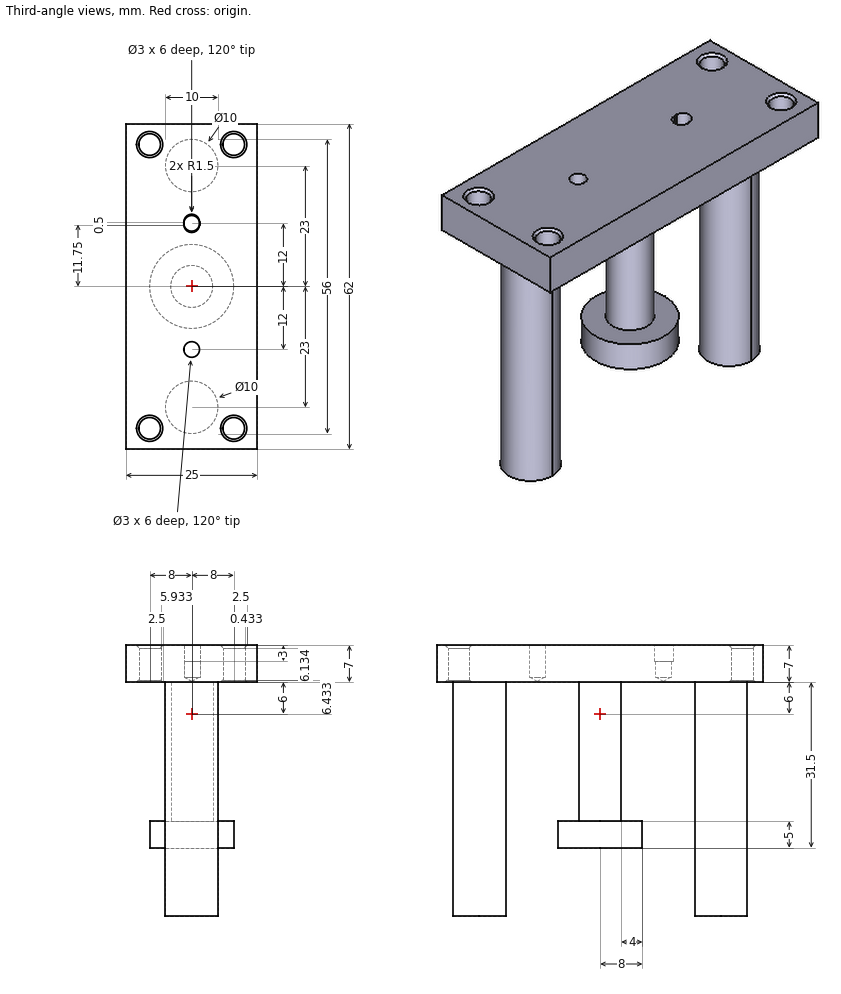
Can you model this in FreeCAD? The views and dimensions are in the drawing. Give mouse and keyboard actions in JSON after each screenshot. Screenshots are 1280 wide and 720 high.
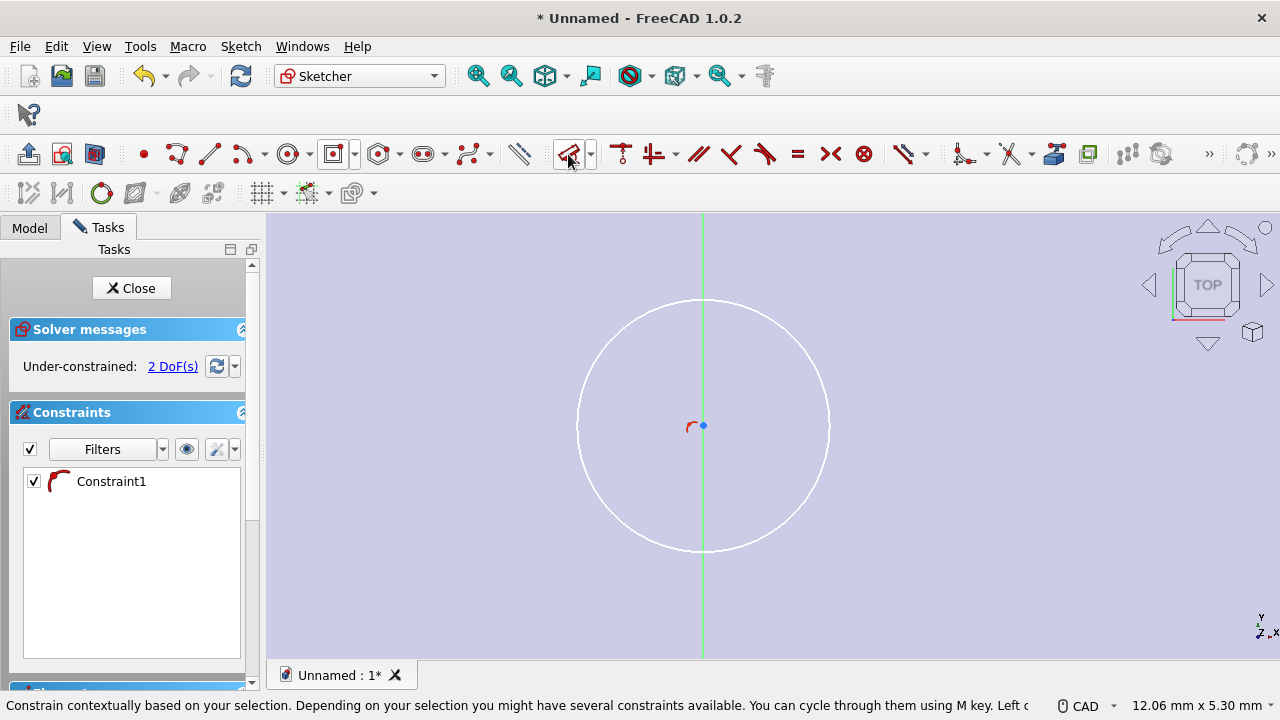
{"action": "left_click", "coordinate": [792, 336]}
{"action": "left_click", "coordinate": [814, 313]}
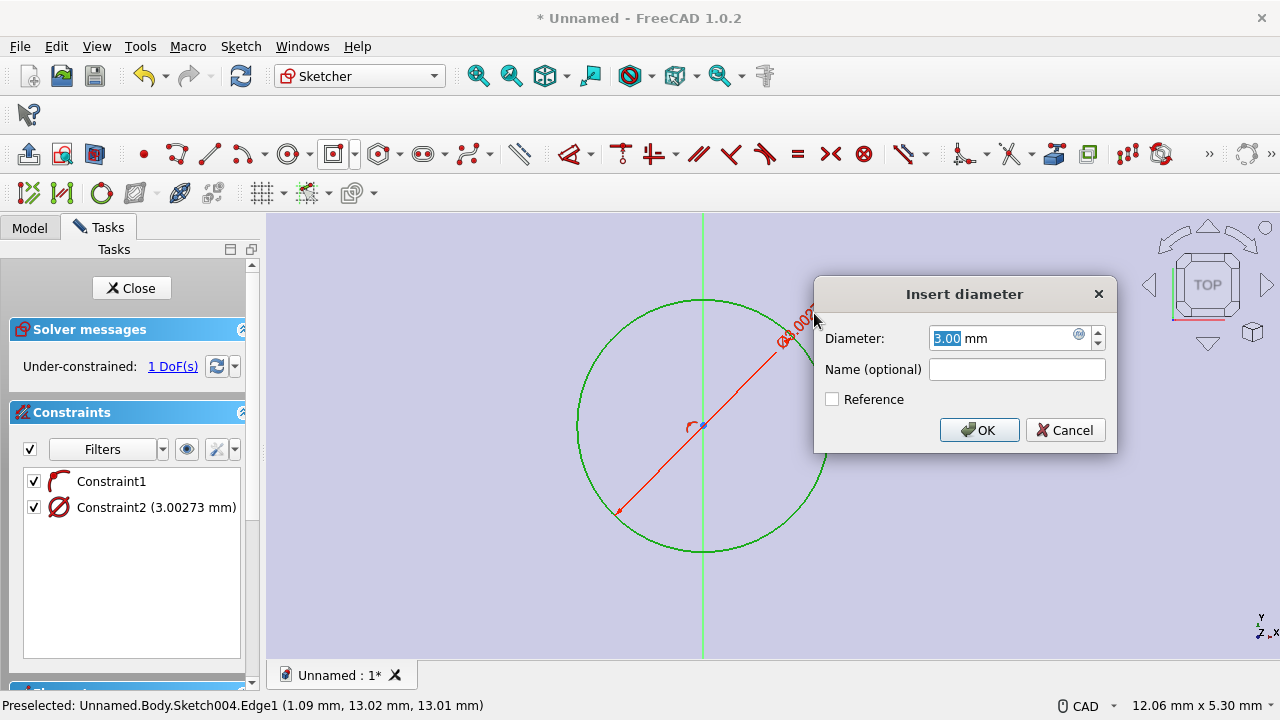
{"action": "type", "text": "3"}
{"action": "key", "text": "Return"}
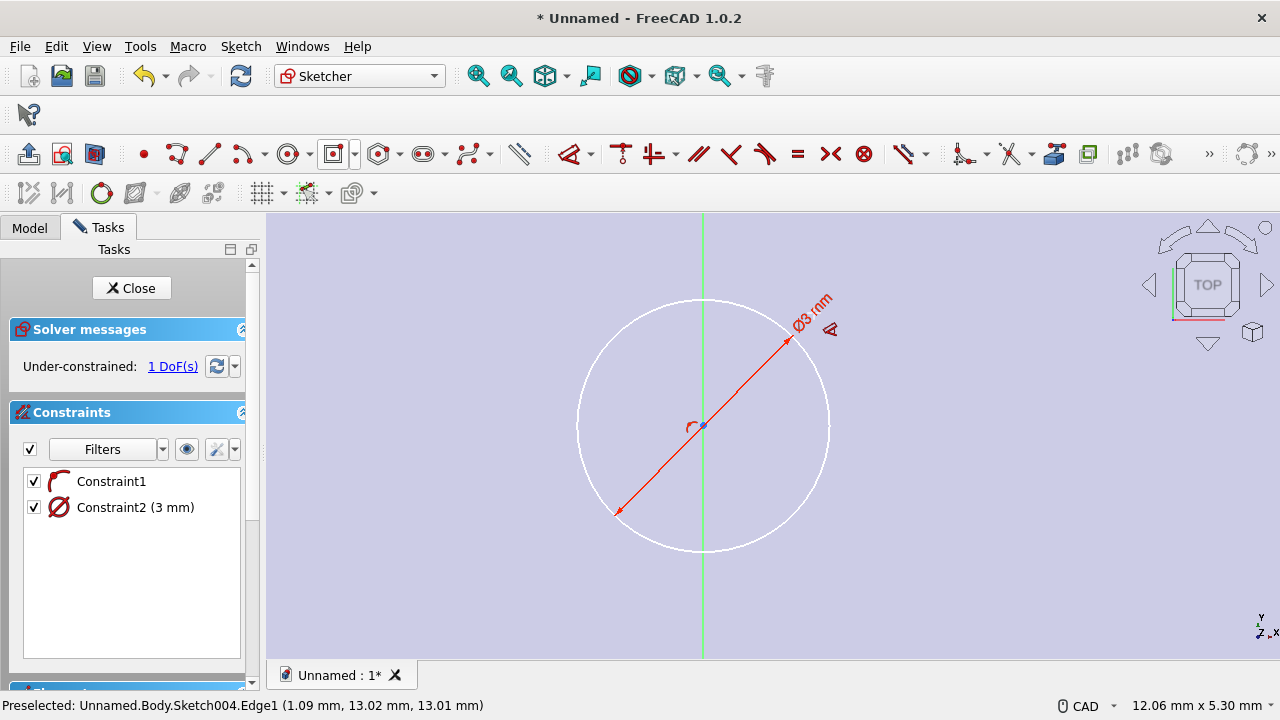
{"action": "left_click", "coordinate": [703, 426]}
{"action": "left_click", "coordinate": [737, 529]}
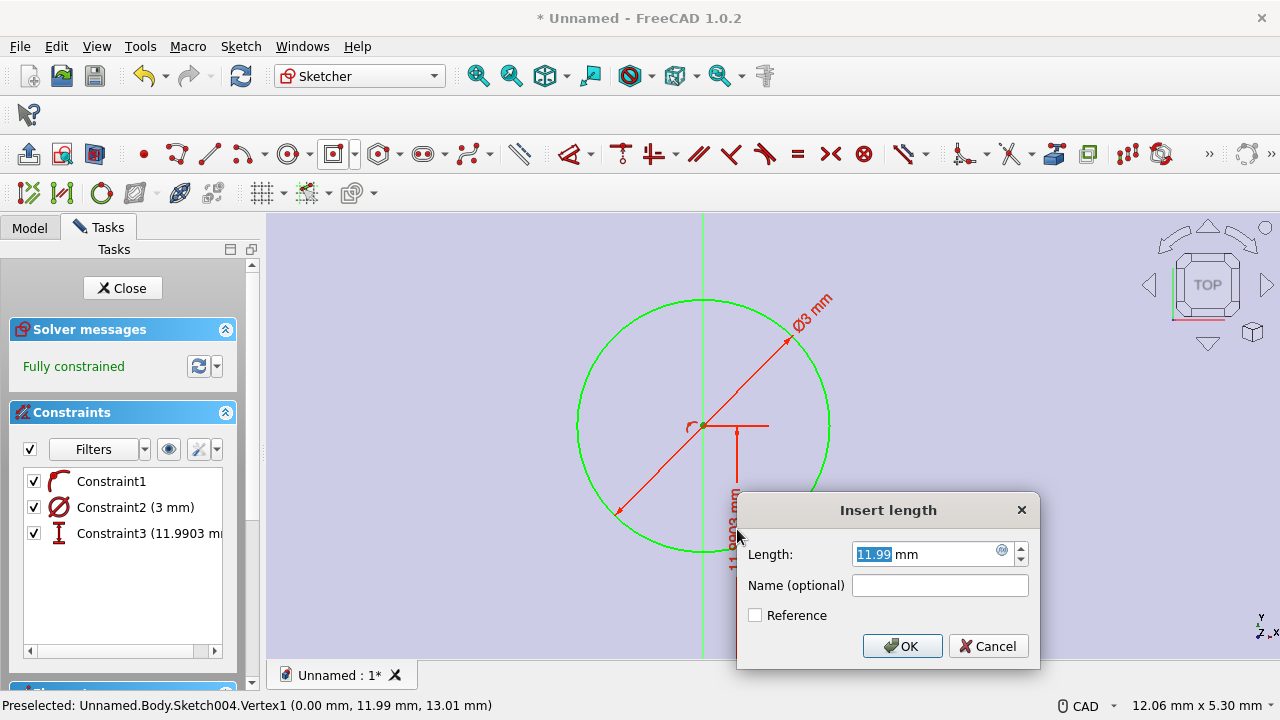
{"action": "type", "text": "12"}
{"action": "key", "text": "Return"}
{"action": "key", "text": "Escape"}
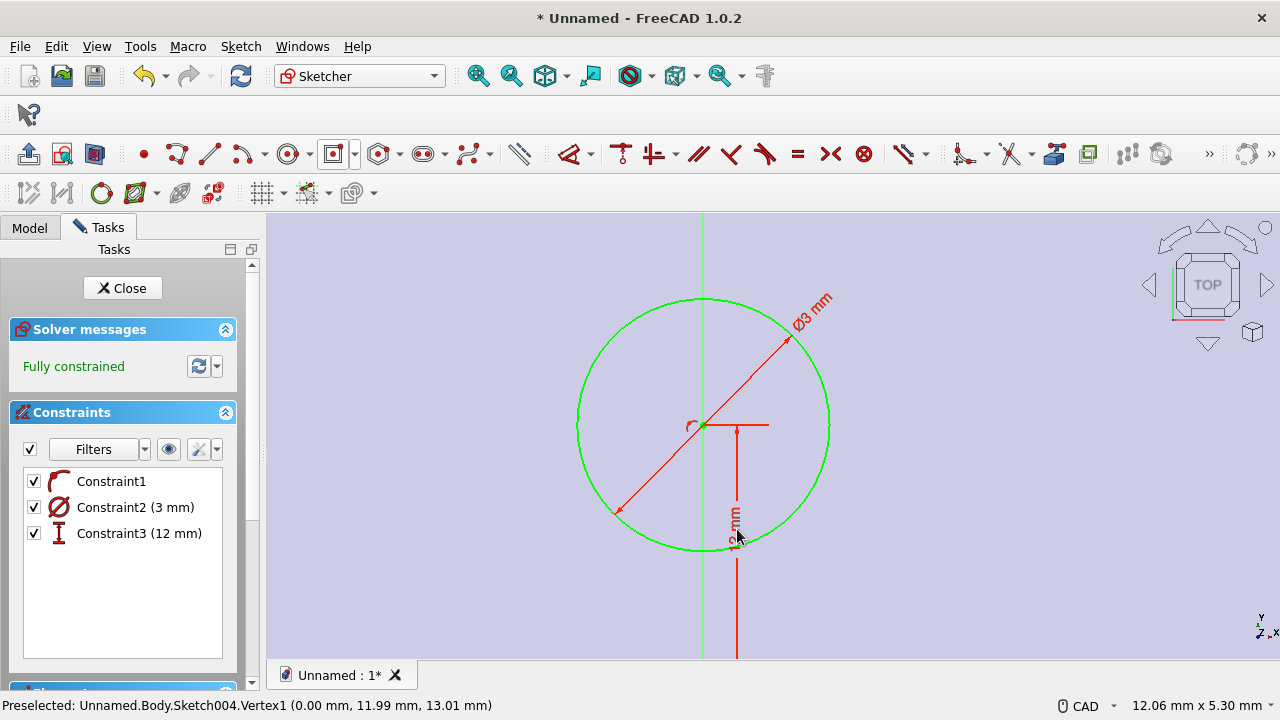
{"action": "left_click", "coordinate": [123, 288]}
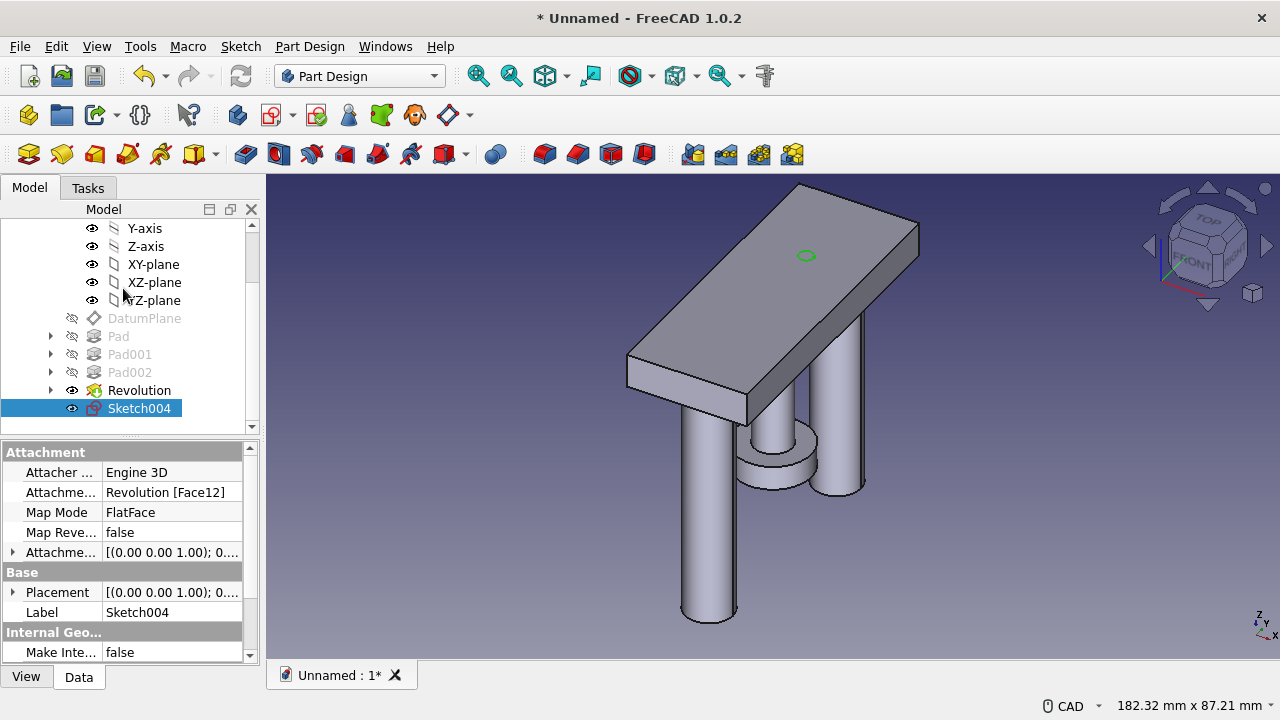
{"action": "left_click", "coordinate": [279, 154]}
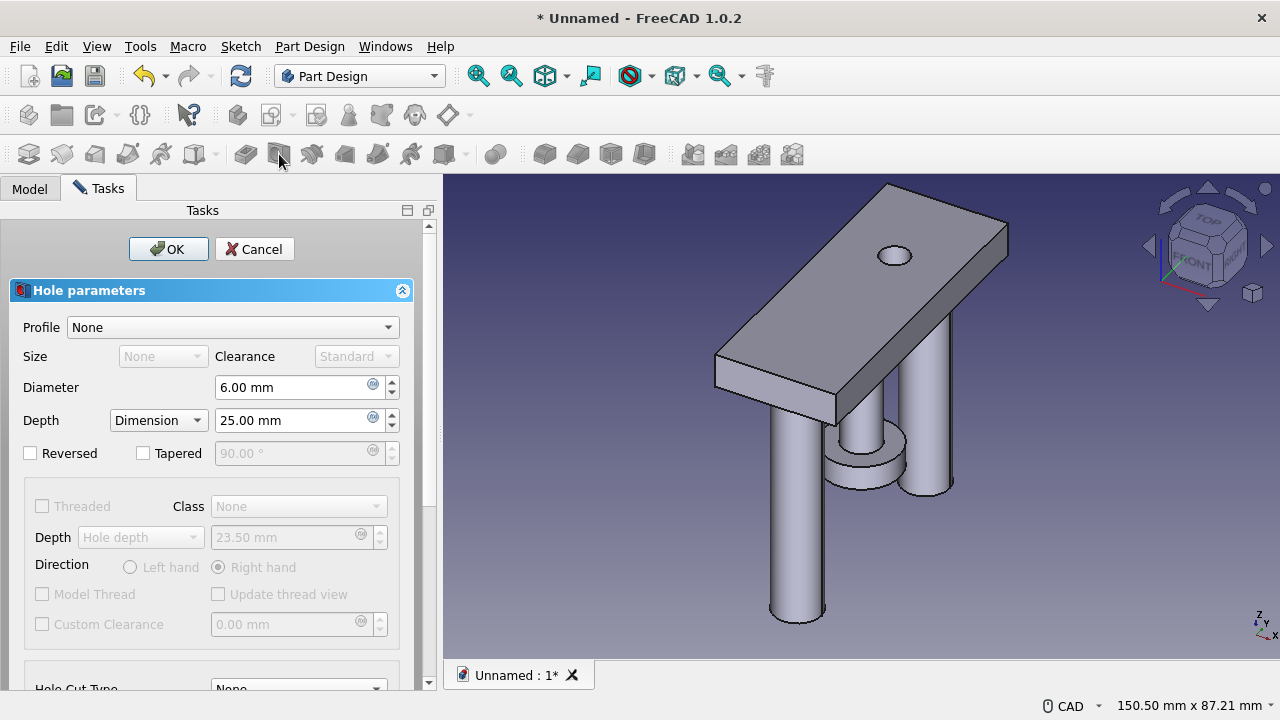
{"action": "triple_click", "coordinate": [300, 388]}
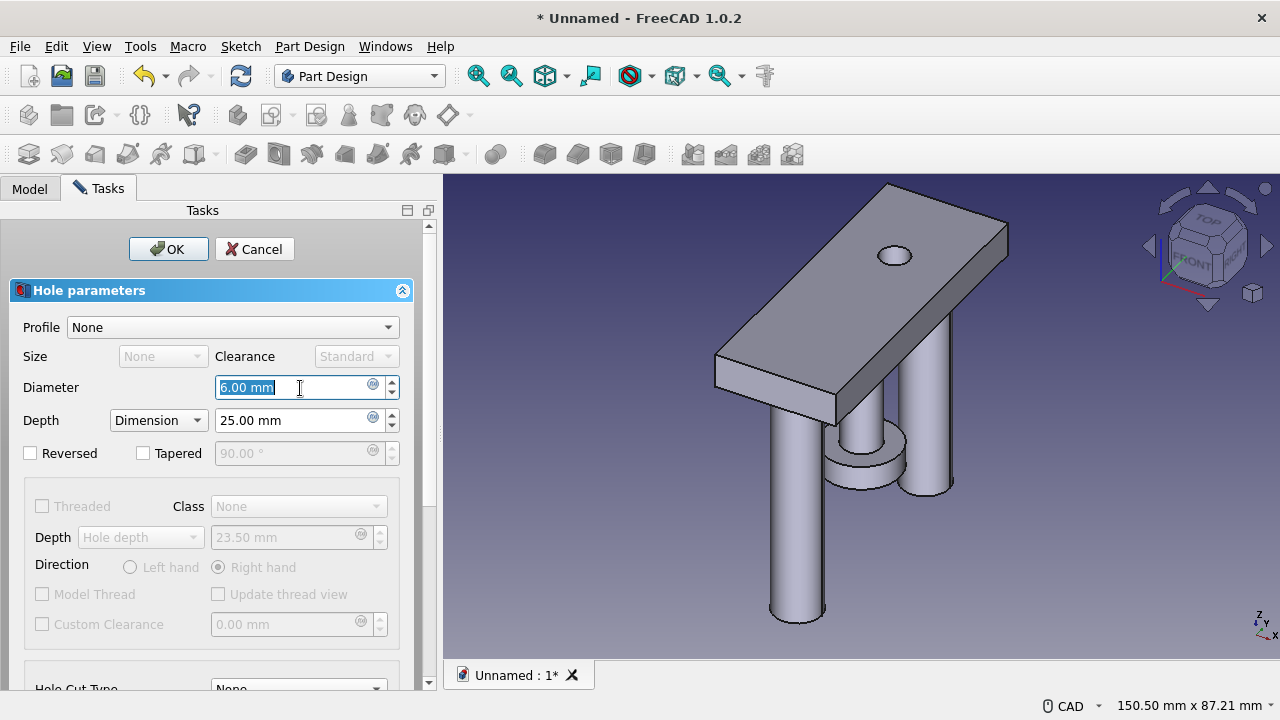
{"action": "type", "text": "3"}
{"action": "key", "text": "Tab"}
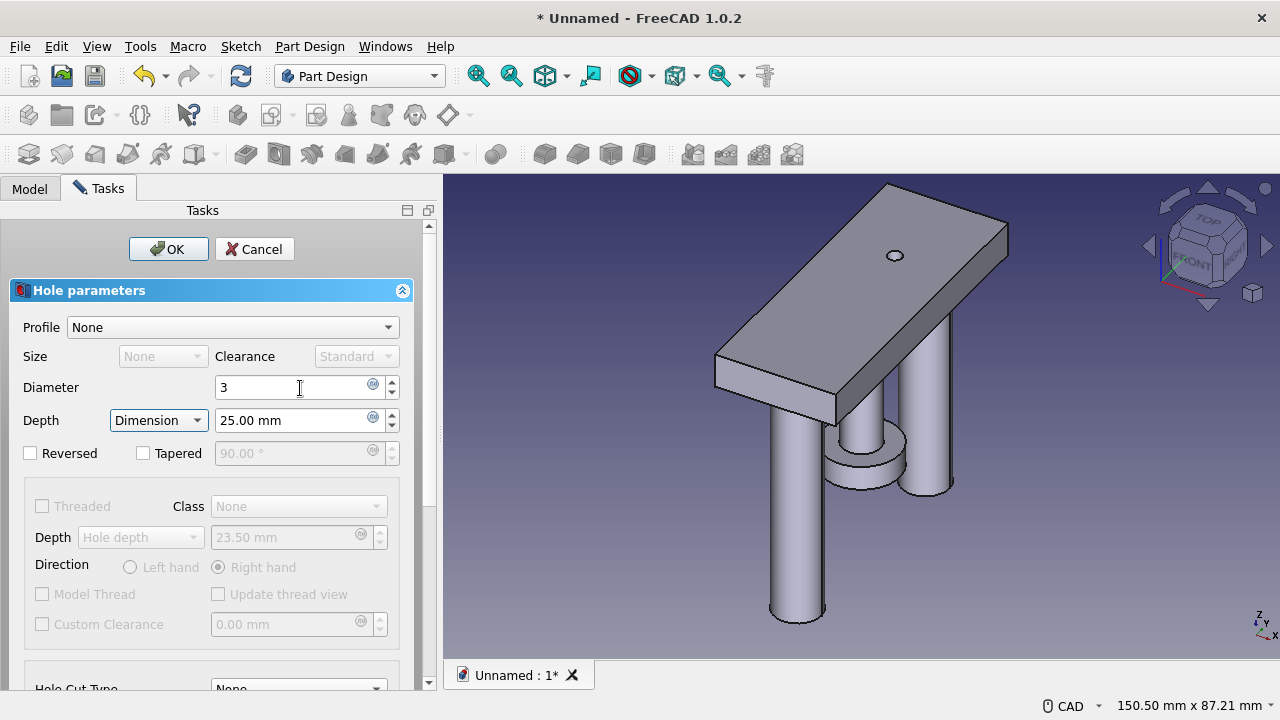
{"action": "triple_click", "coordinate": [300, 420]}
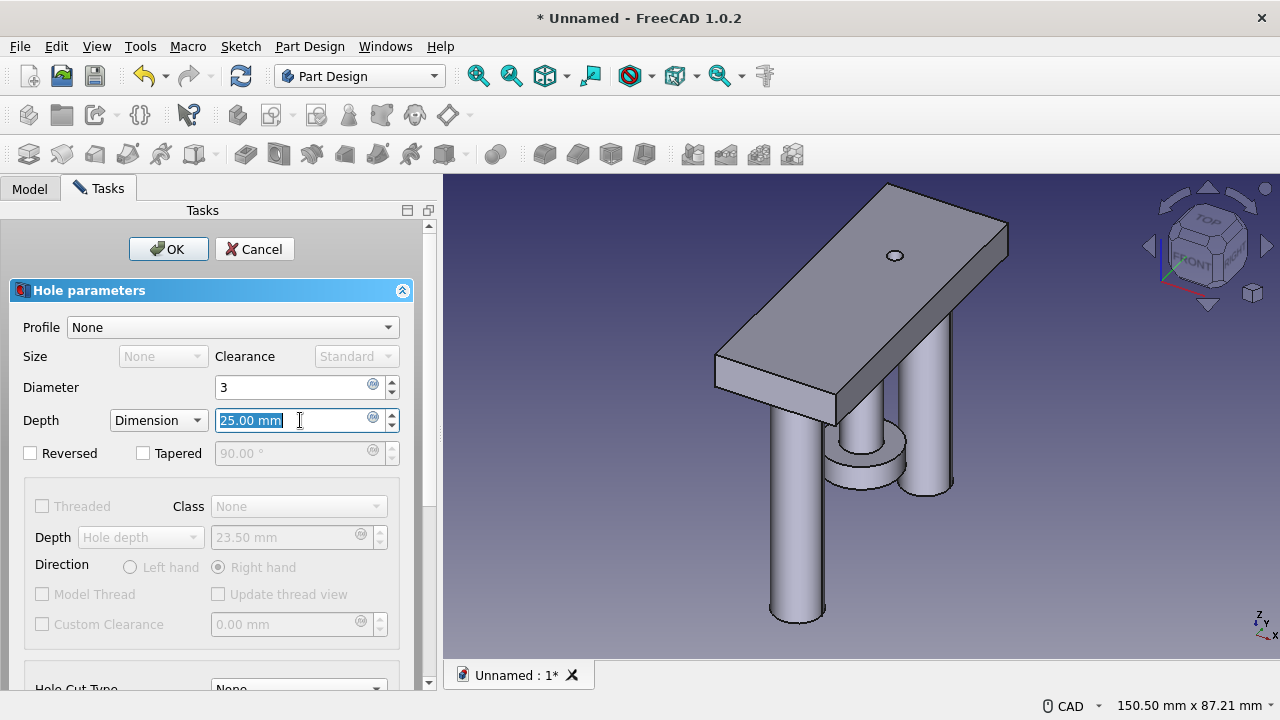
{"action": "type", "text": "6"}
{"action": "key", "text": "Tab"}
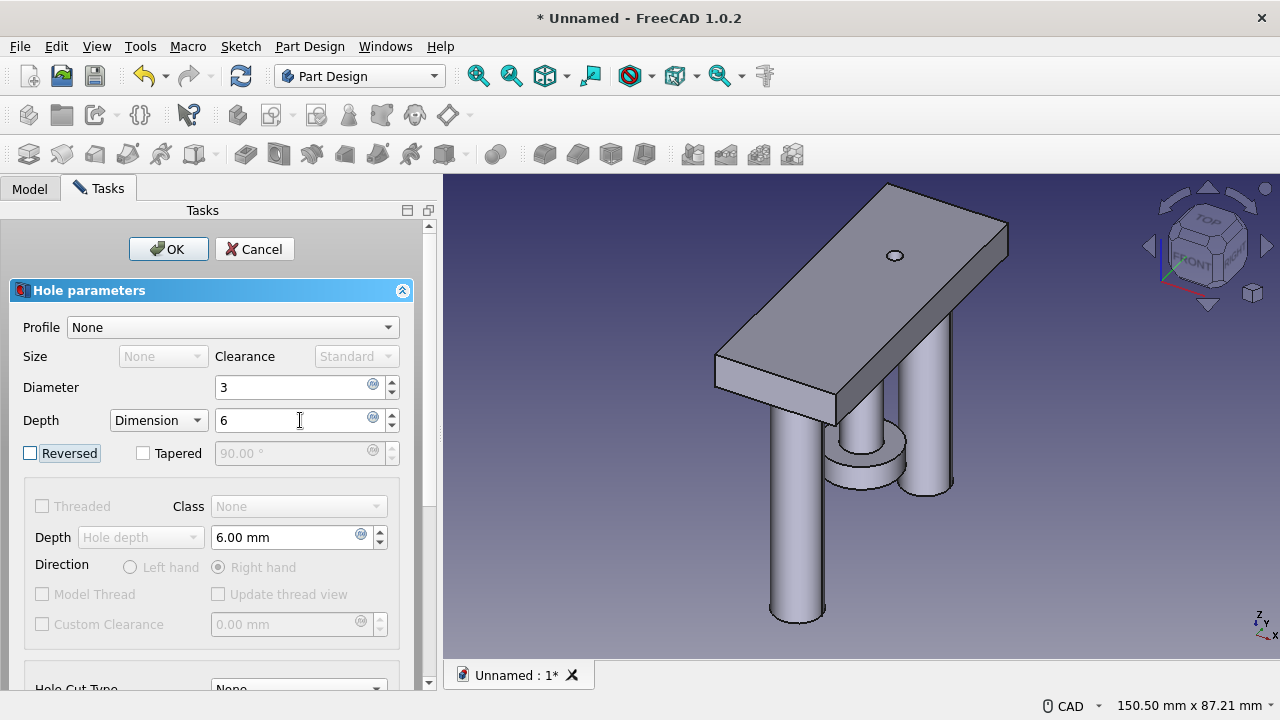
{"action": "scroll", "coordinate": [429, 455], "scroll_direction": "down", "scroll_amount": 5}